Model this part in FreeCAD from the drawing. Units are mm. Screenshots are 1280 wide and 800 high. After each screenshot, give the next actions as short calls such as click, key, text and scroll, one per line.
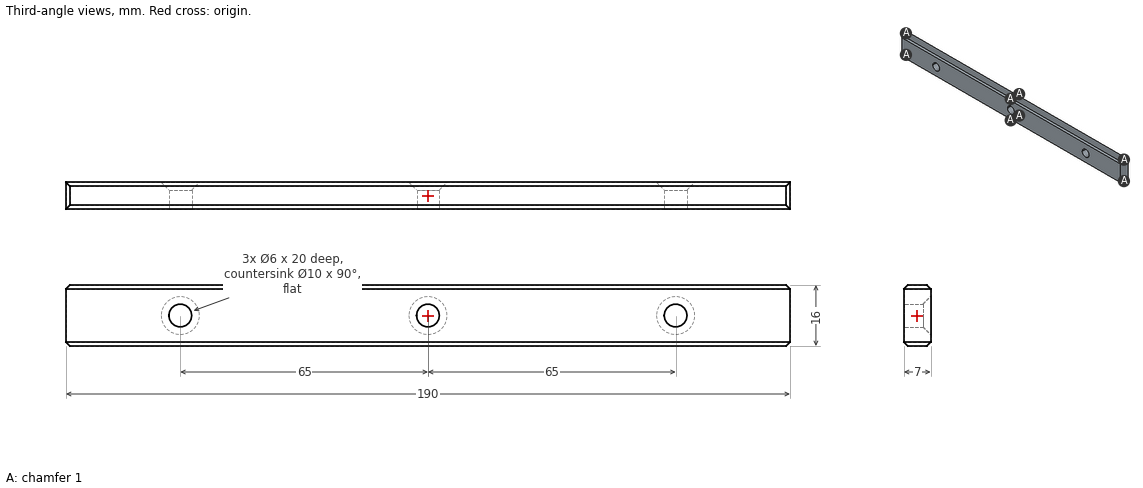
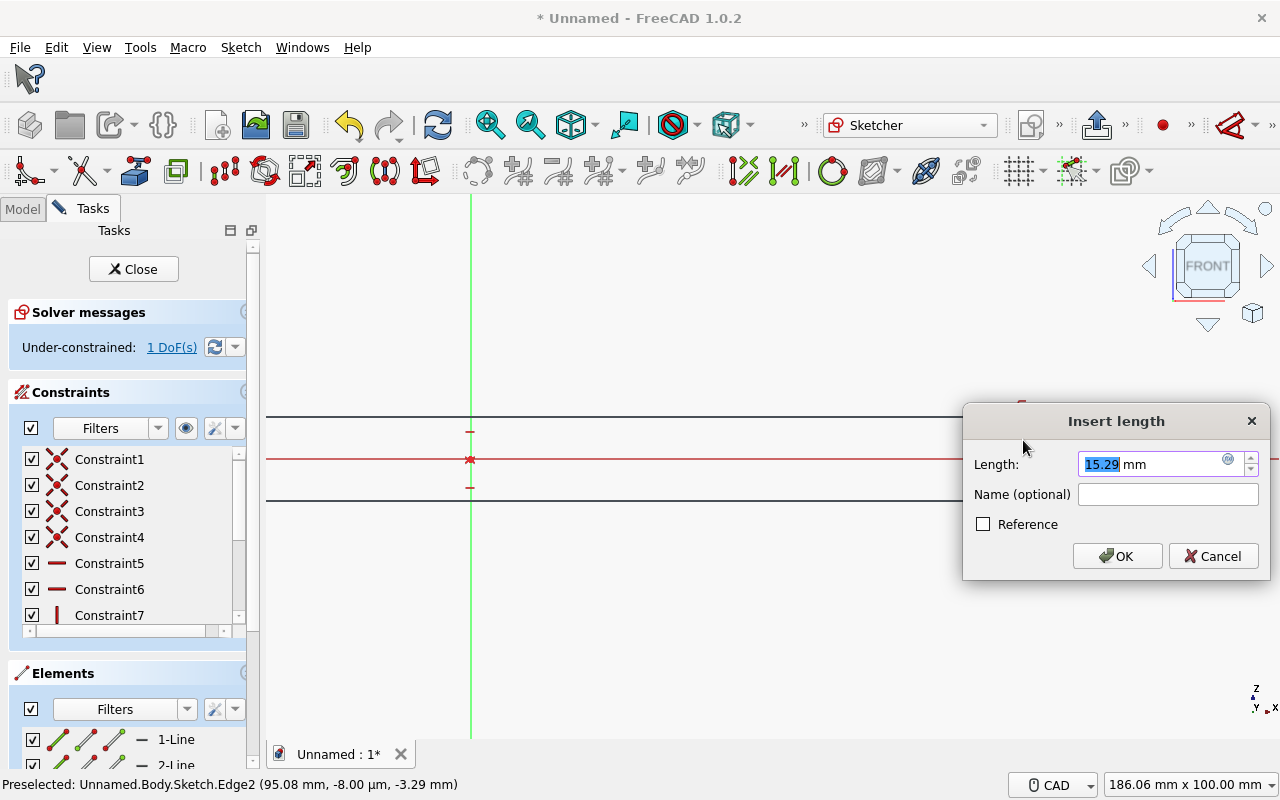
text(16)
key(Return)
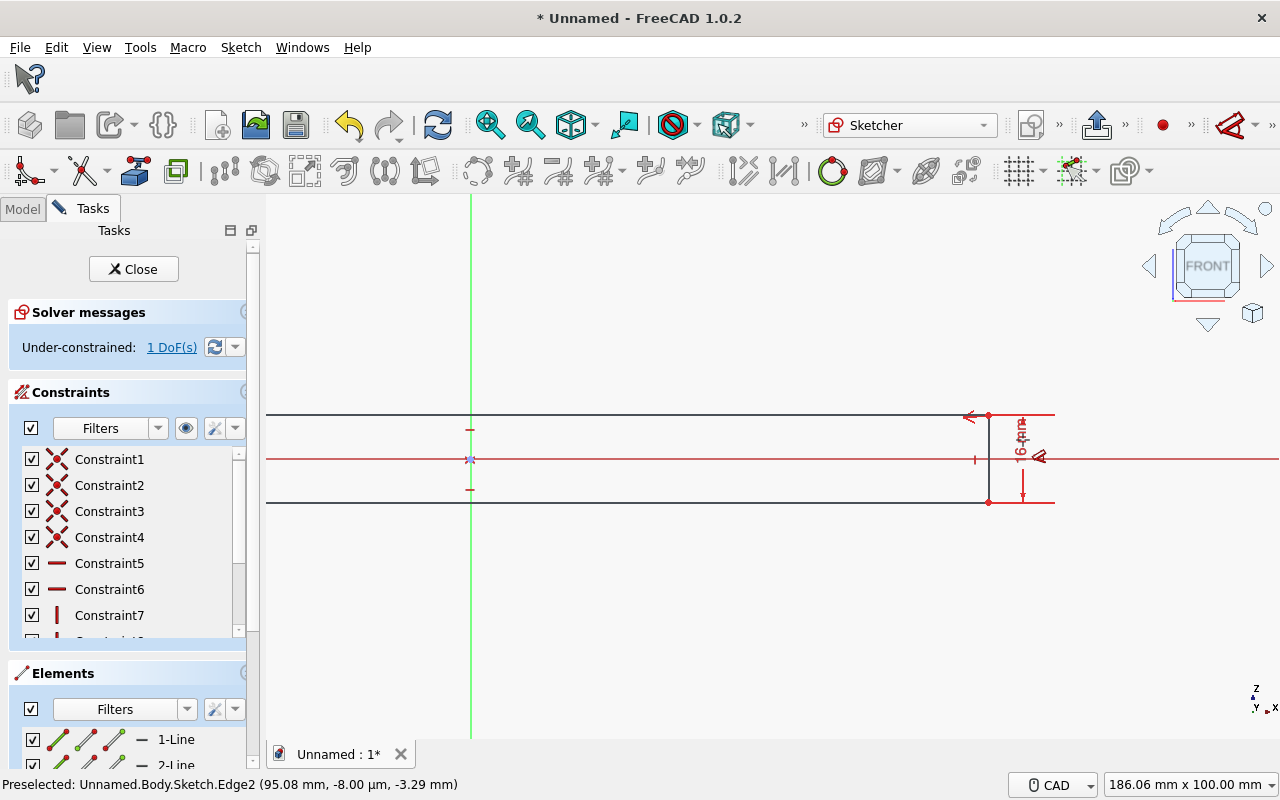
click(678, 503)
click(641, 537)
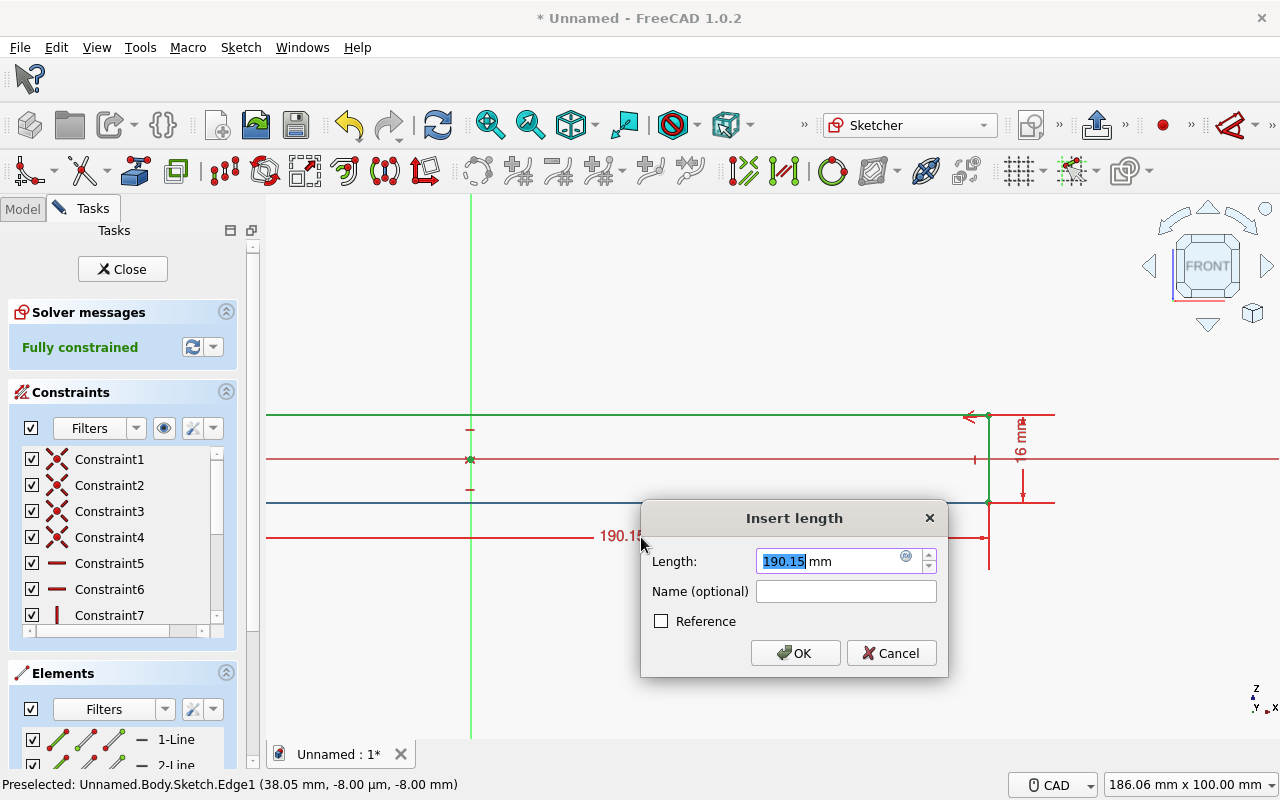
text(190)
key(Return)
key(Escape)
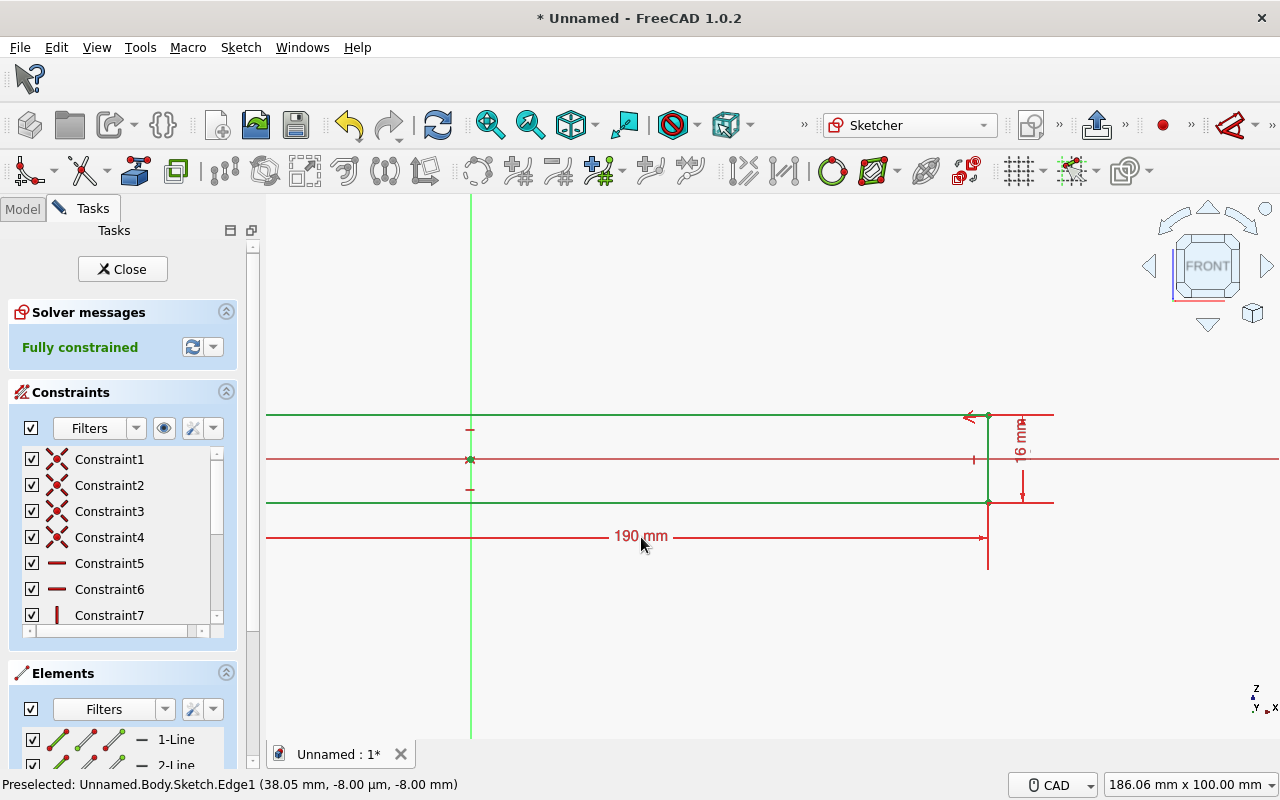
click(123, 269)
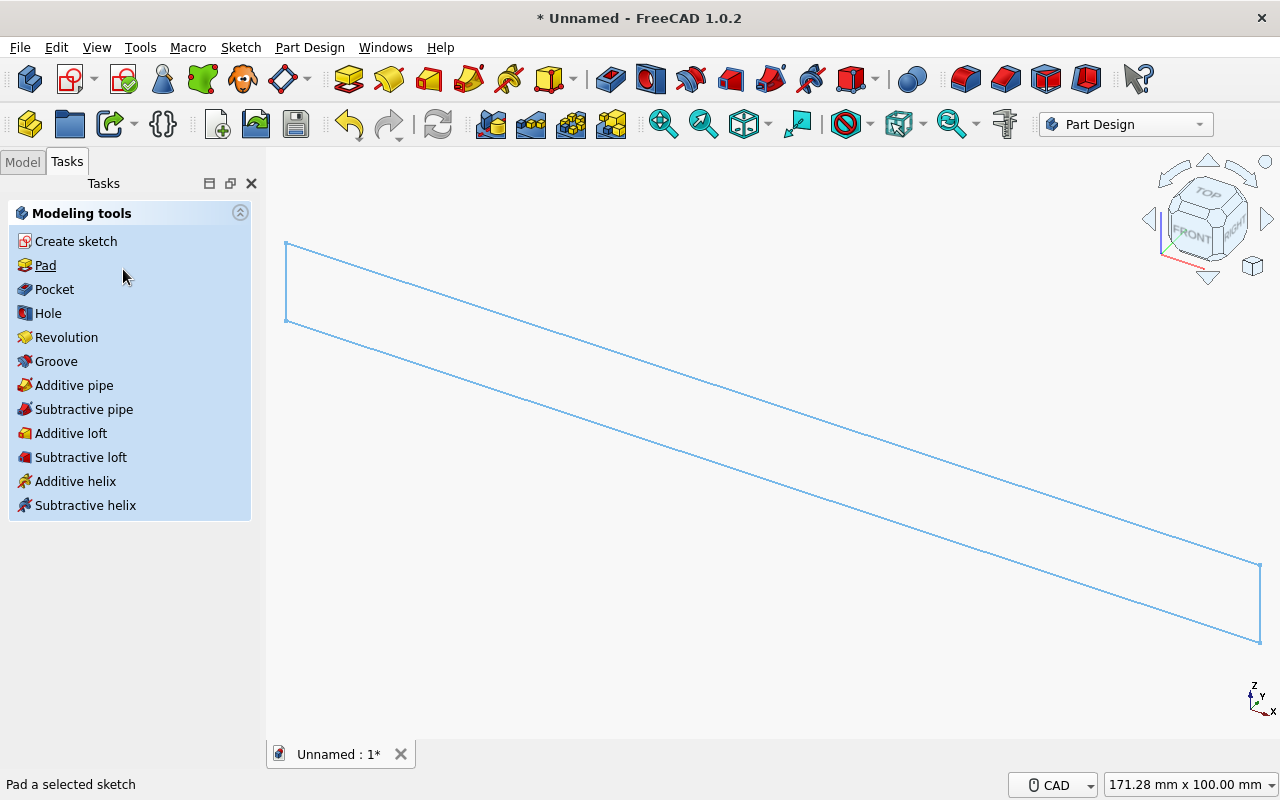
click(350, 80)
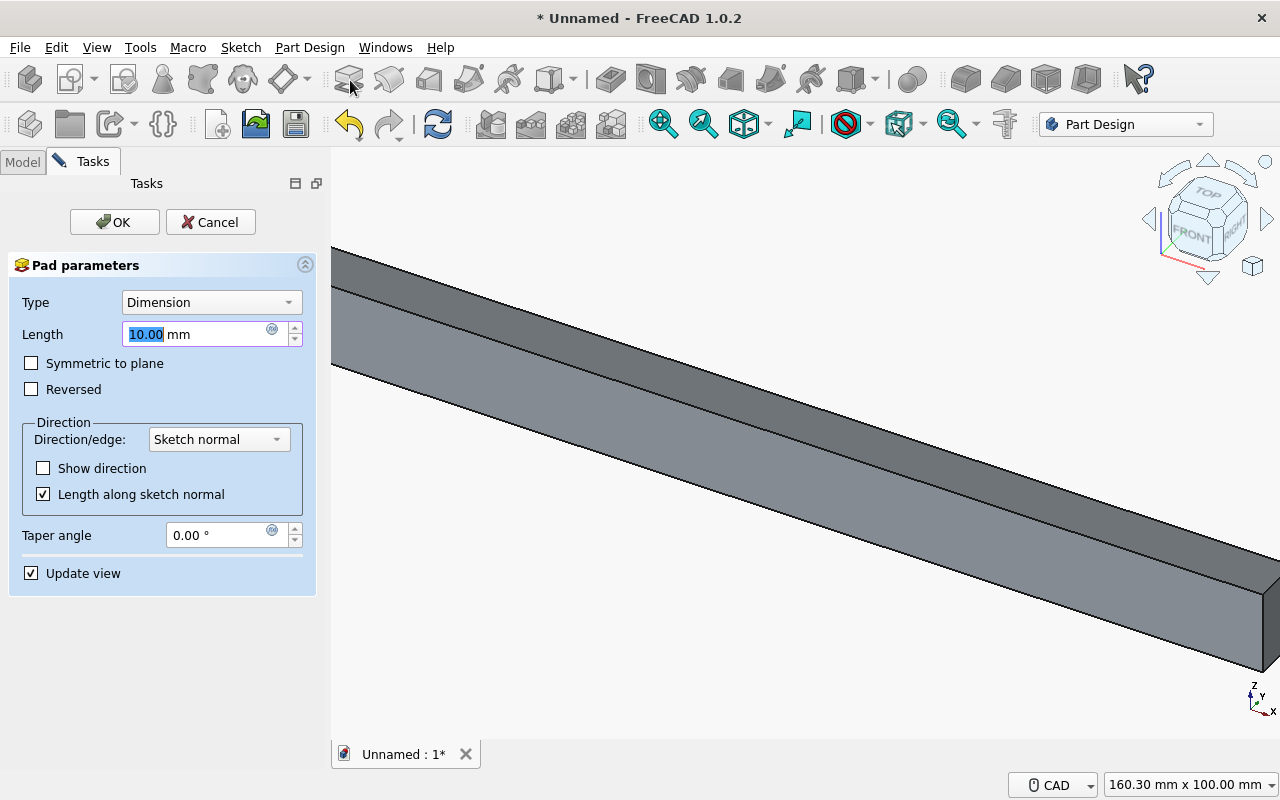
text(7)
key(Tab)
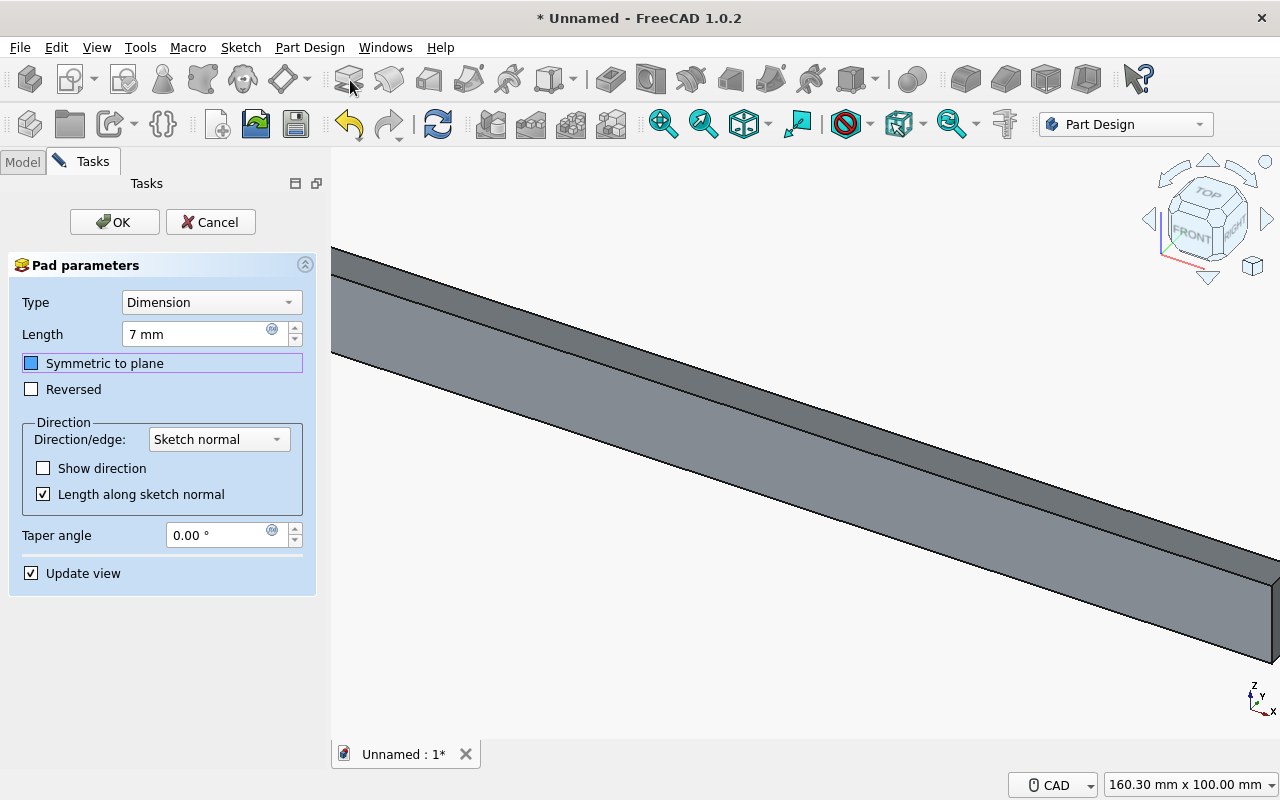
click(30, 363)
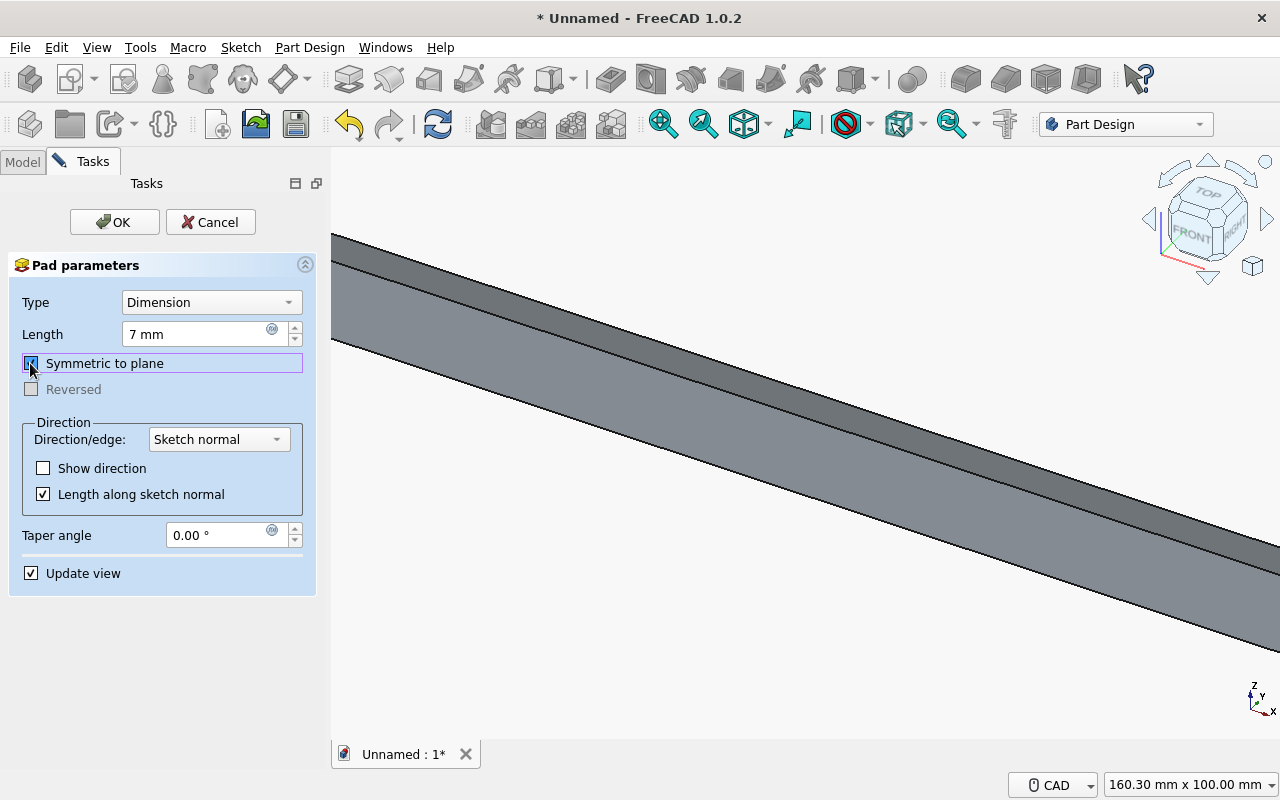
click(115, 222)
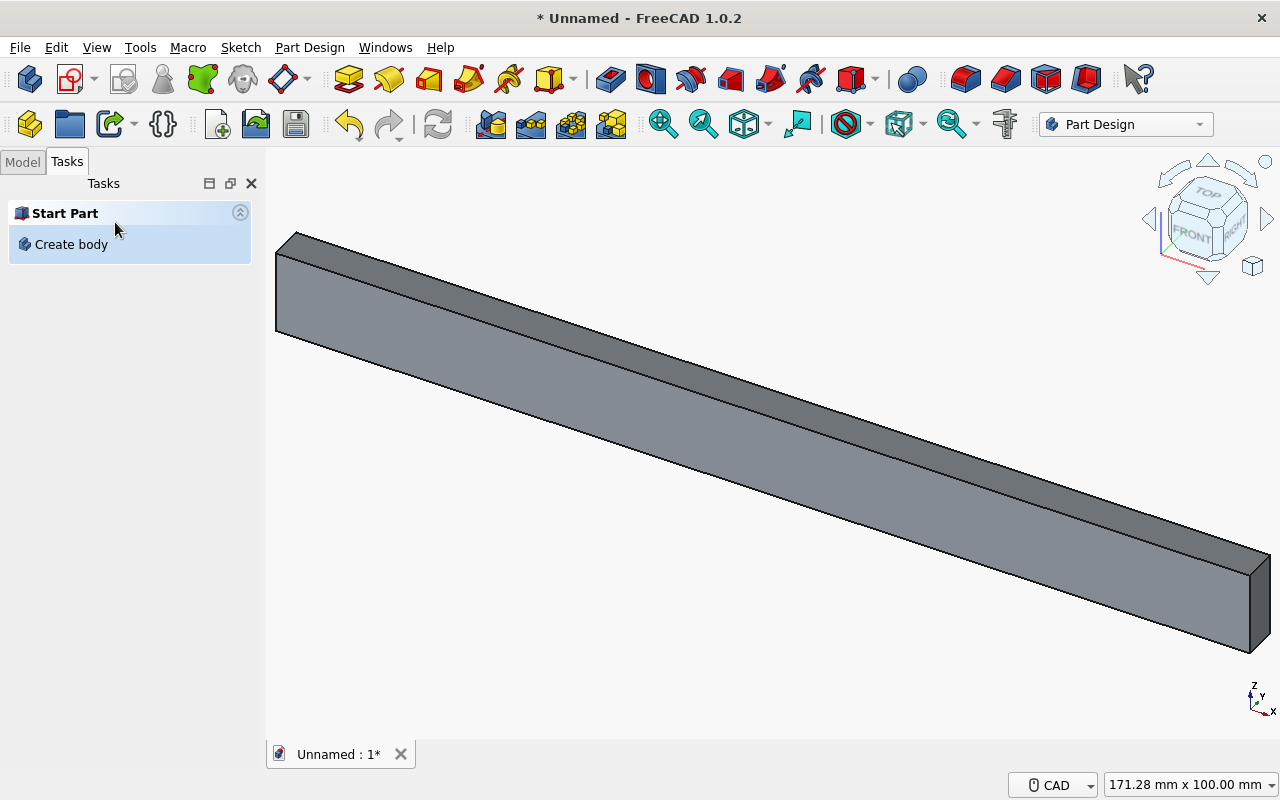
key(4)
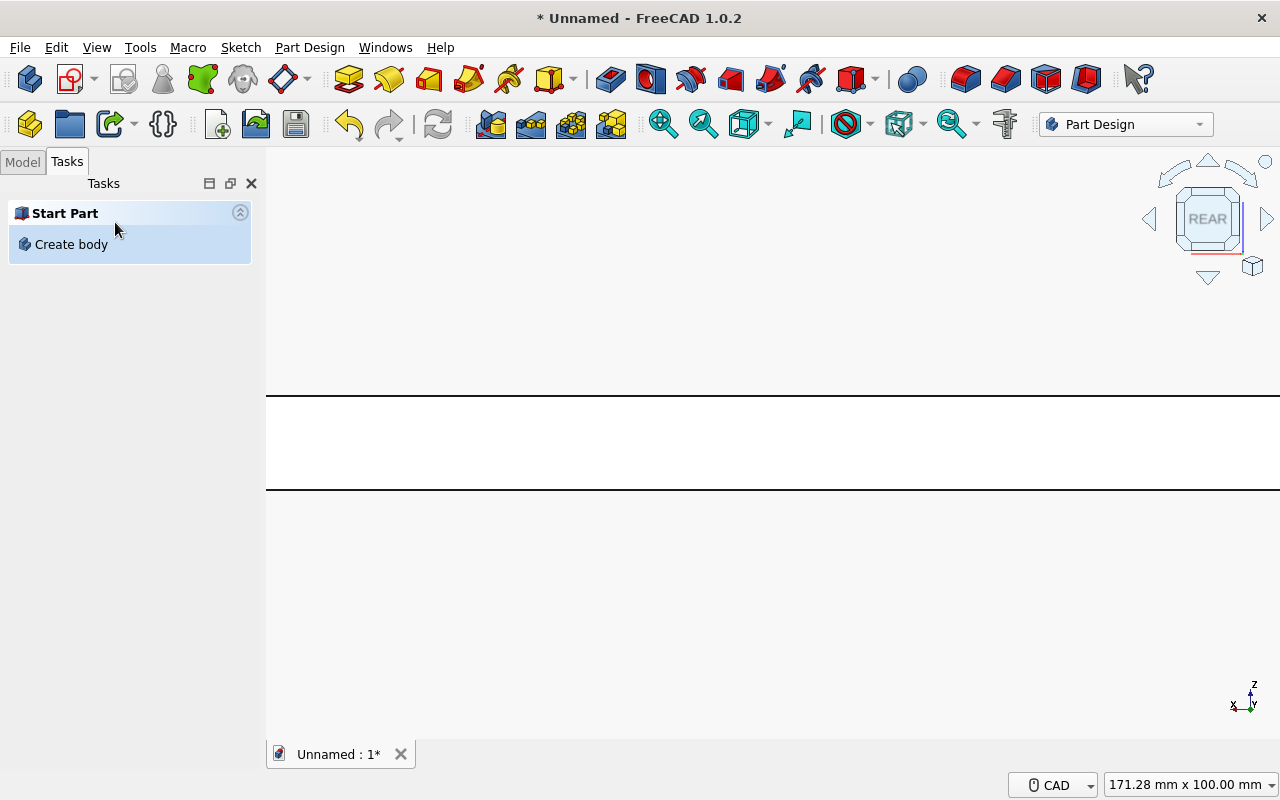
click(664, 124)